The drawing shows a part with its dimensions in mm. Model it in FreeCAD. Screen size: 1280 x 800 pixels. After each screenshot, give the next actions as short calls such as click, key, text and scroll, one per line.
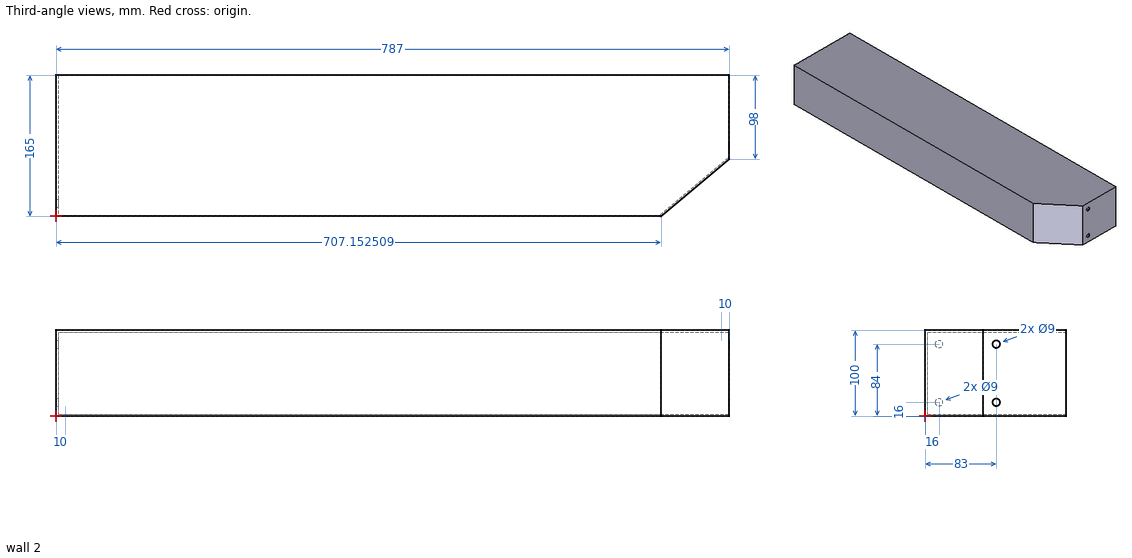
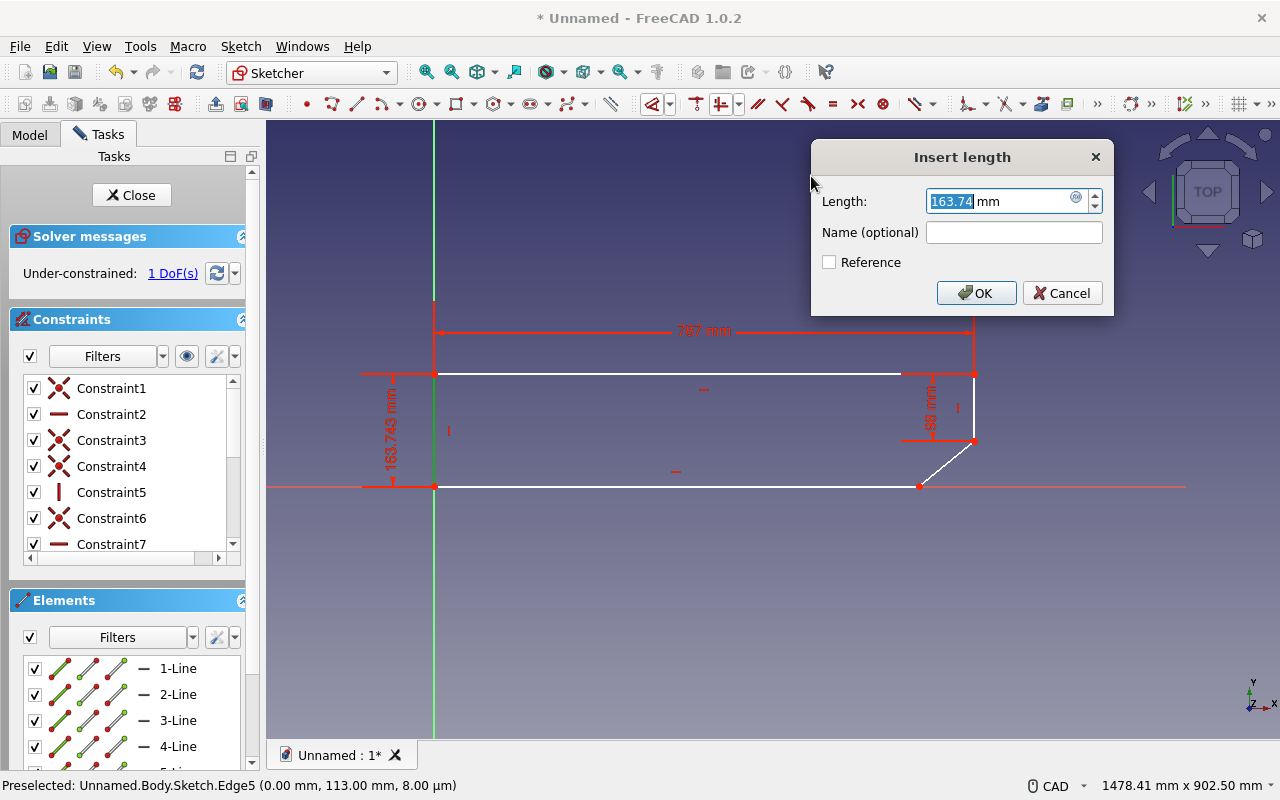
text(165)
key(Return)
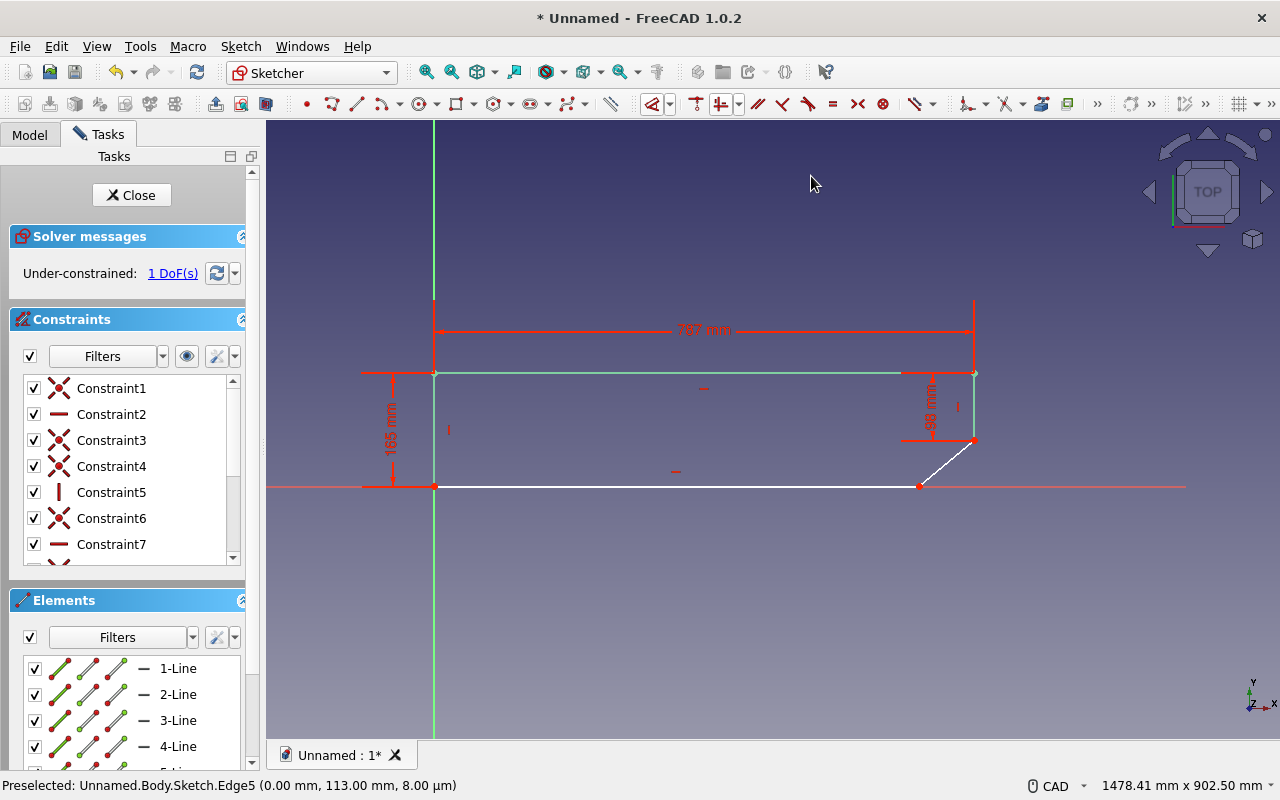
click(580, 487)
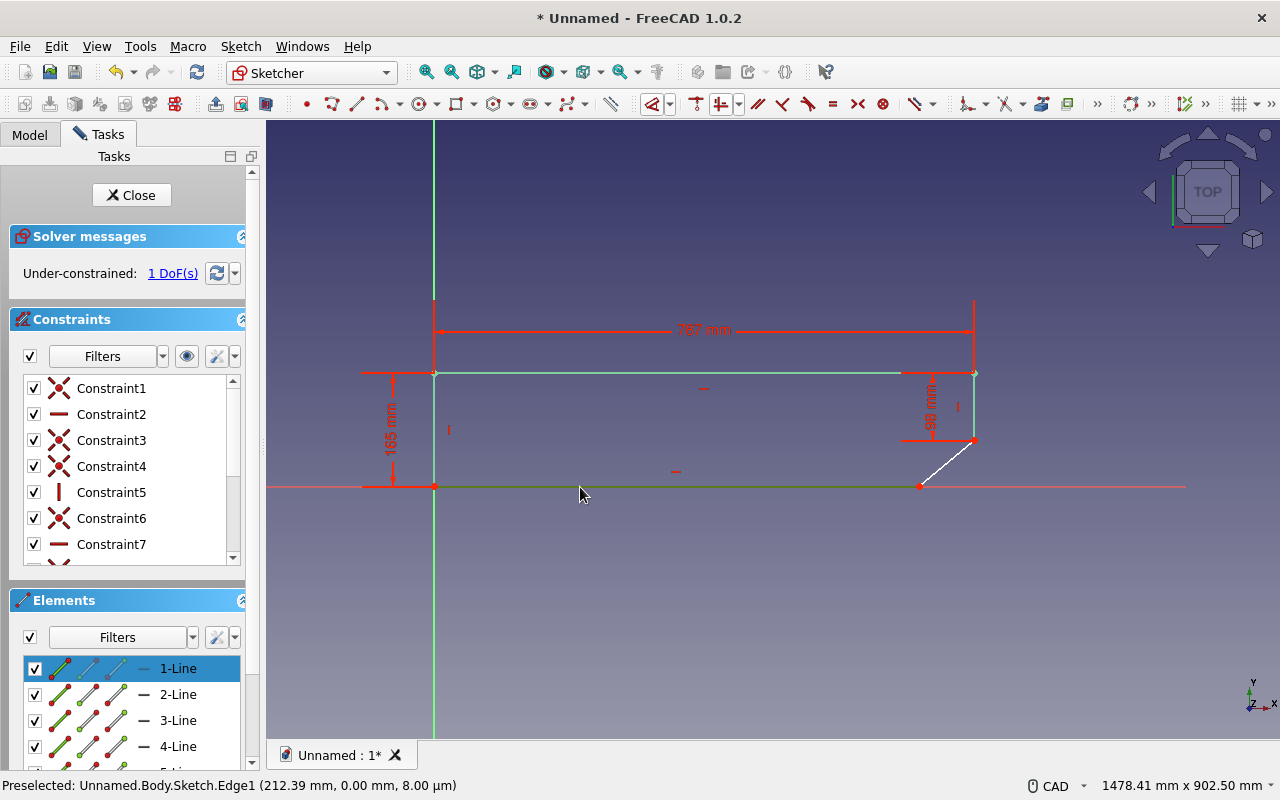
key(l)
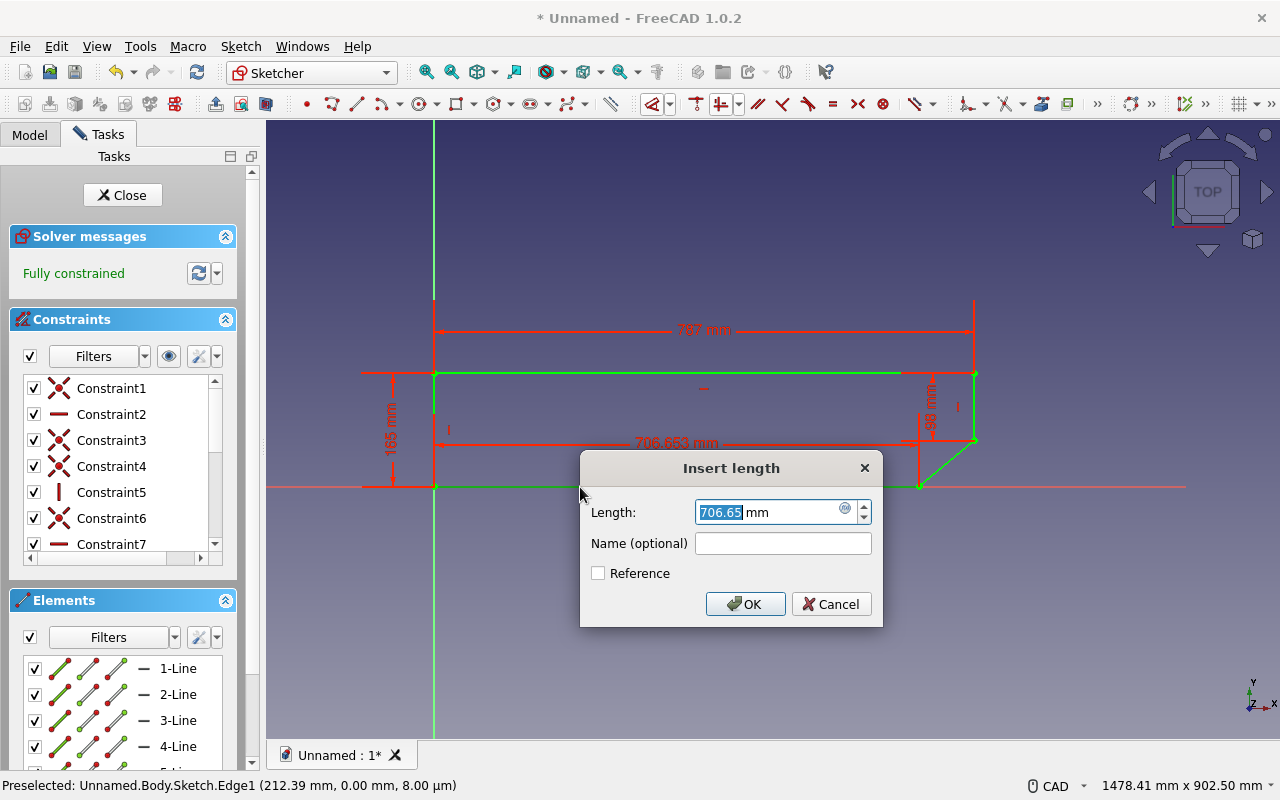
text(707.152509)
key(Return)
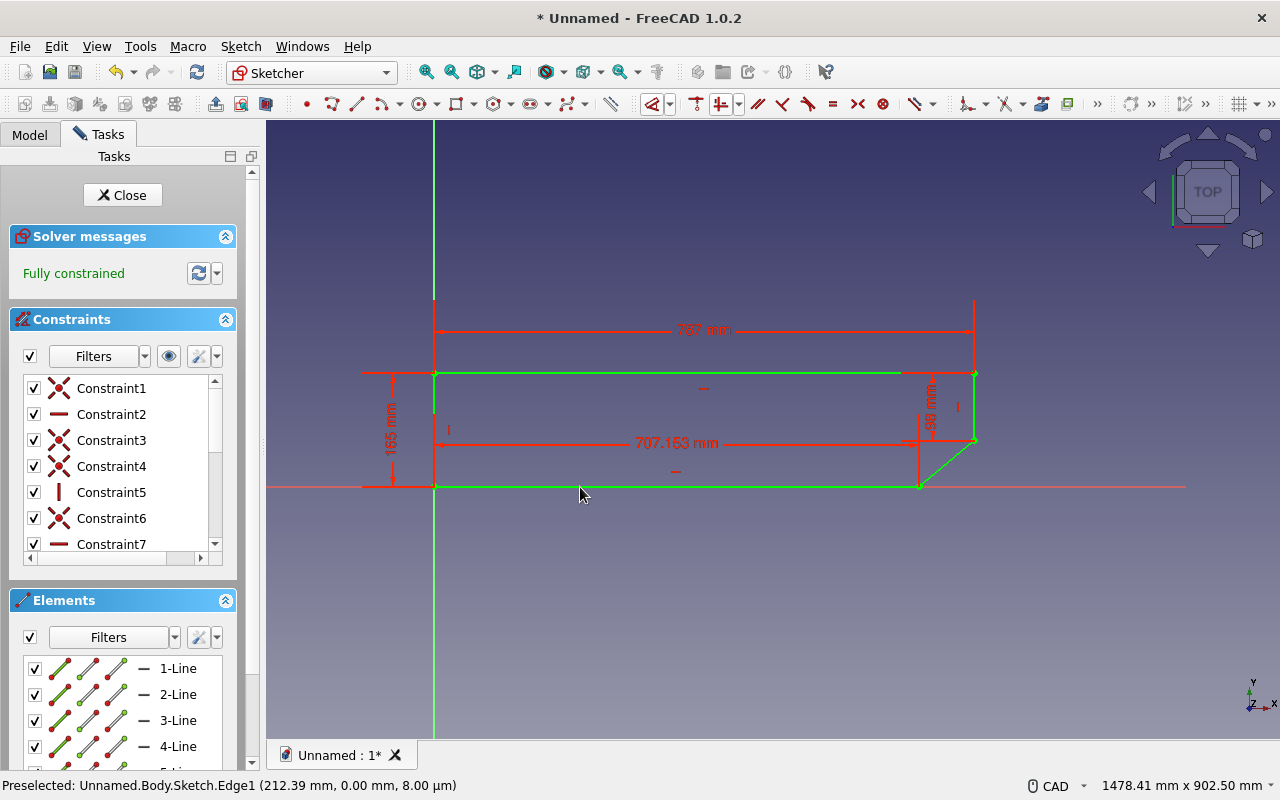
click(123, 195)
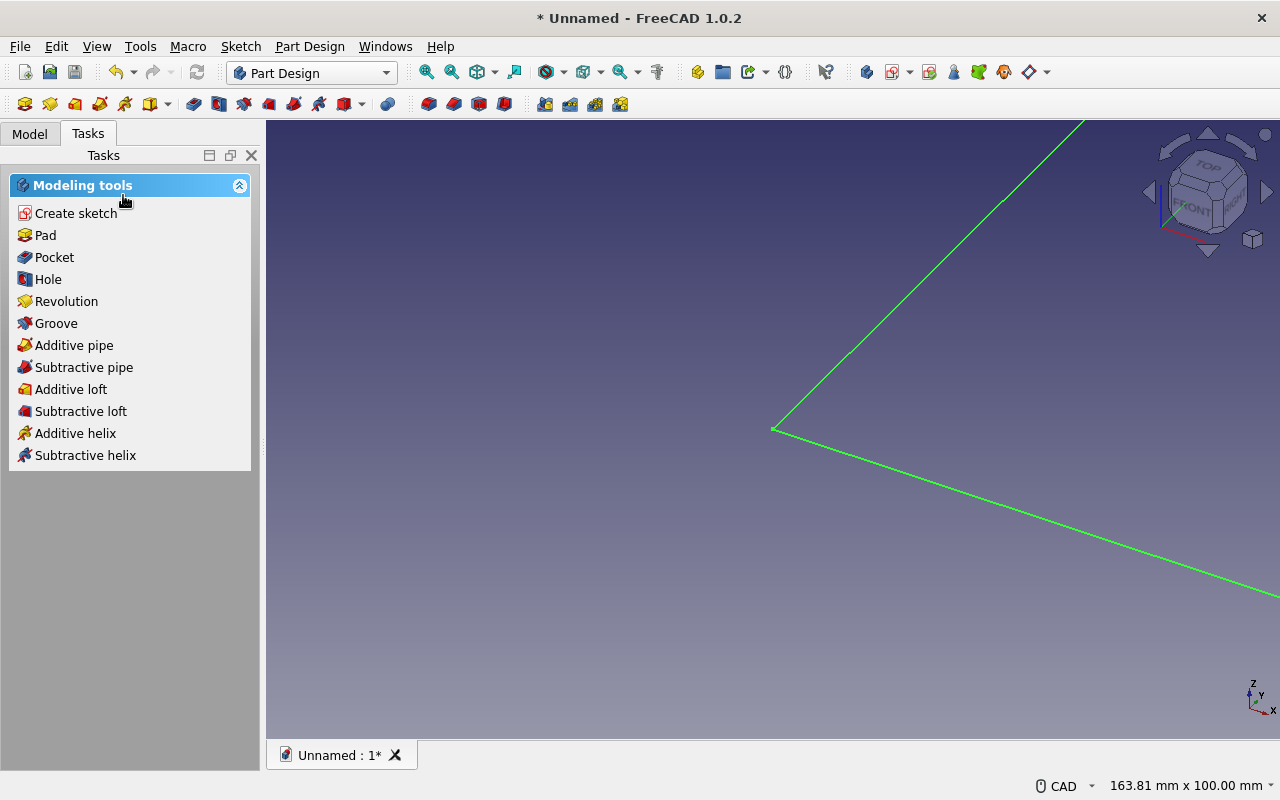
click(25, 104)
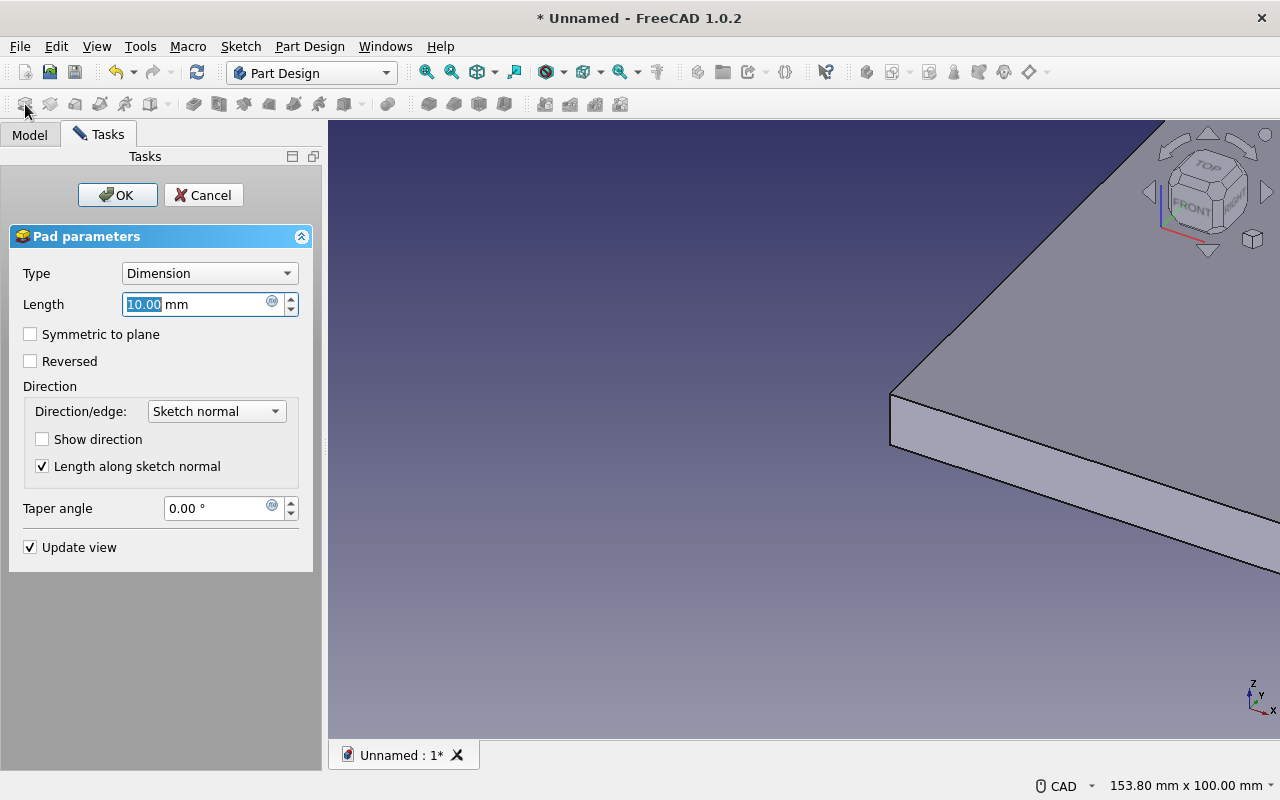
text(100)
key(Tab)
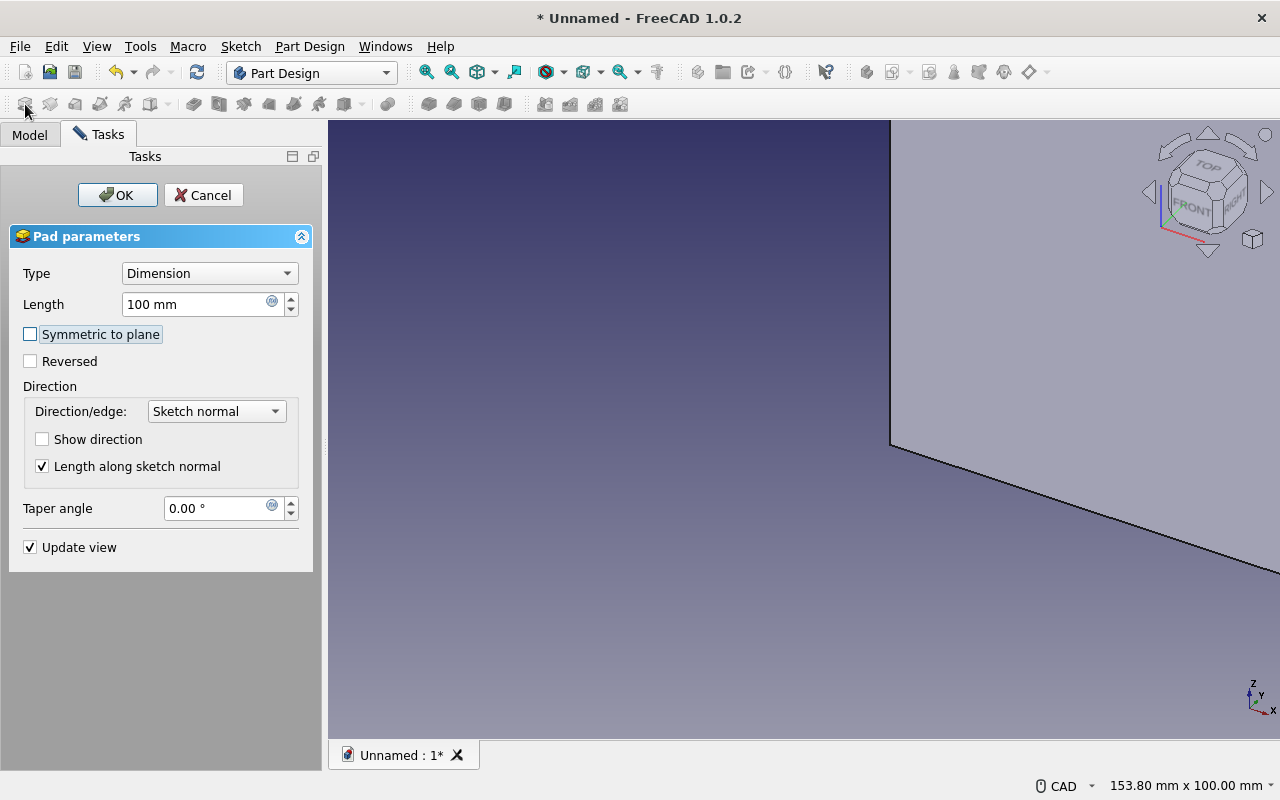
click(118, 195)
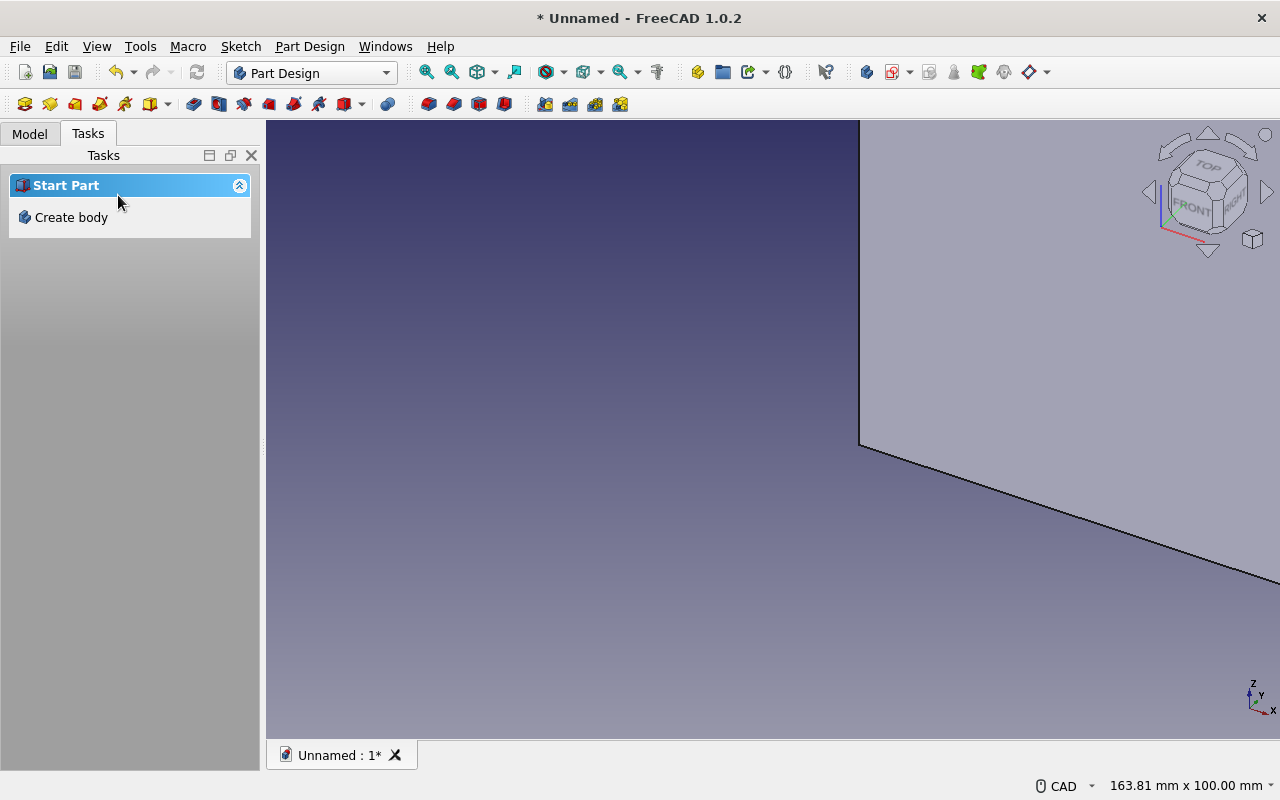
click(427, 72)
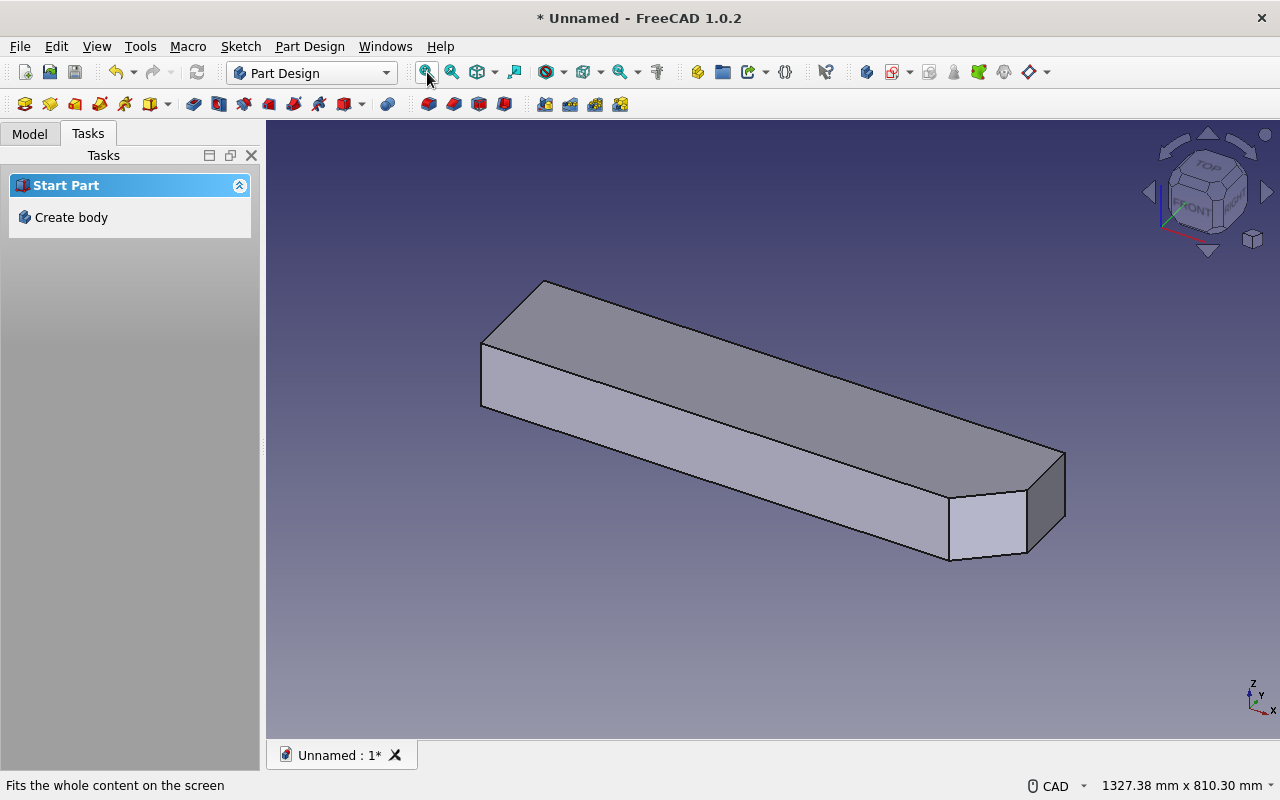
key(0)